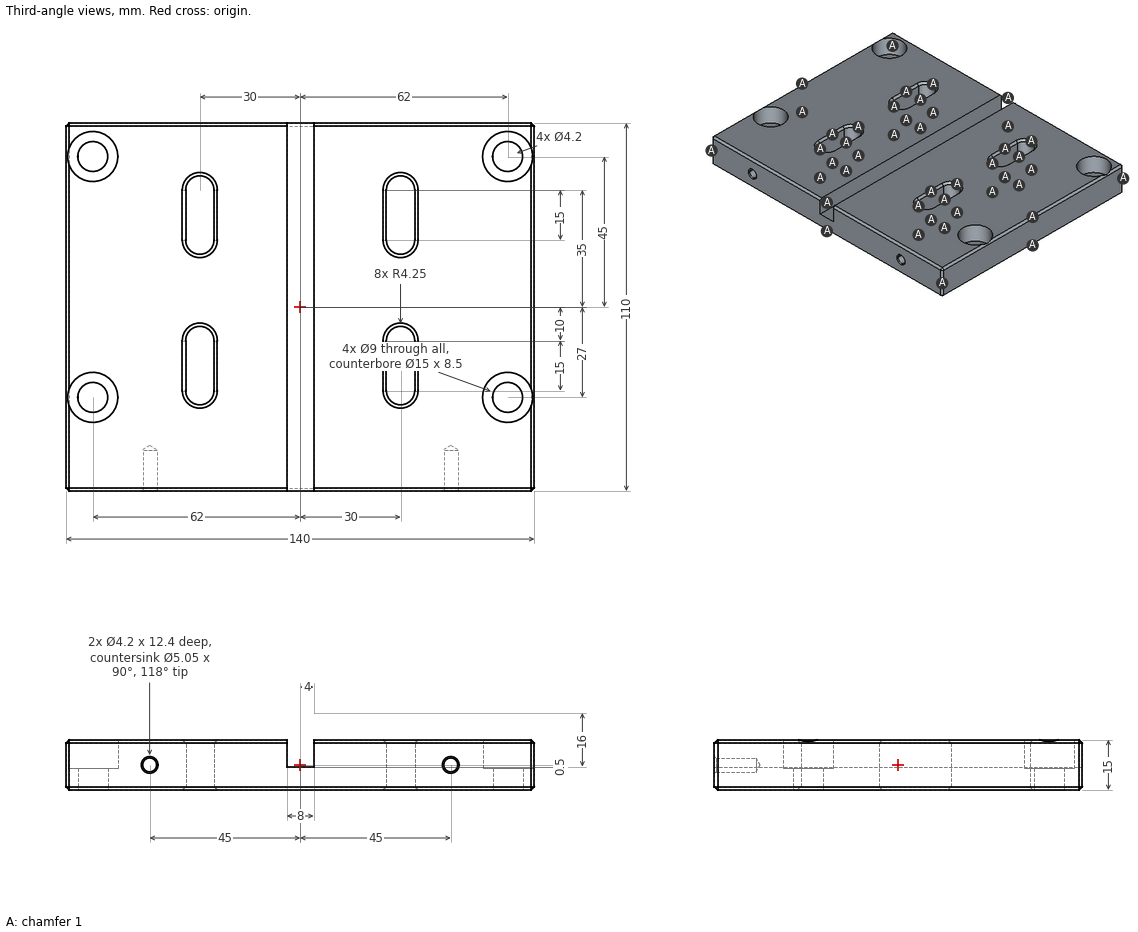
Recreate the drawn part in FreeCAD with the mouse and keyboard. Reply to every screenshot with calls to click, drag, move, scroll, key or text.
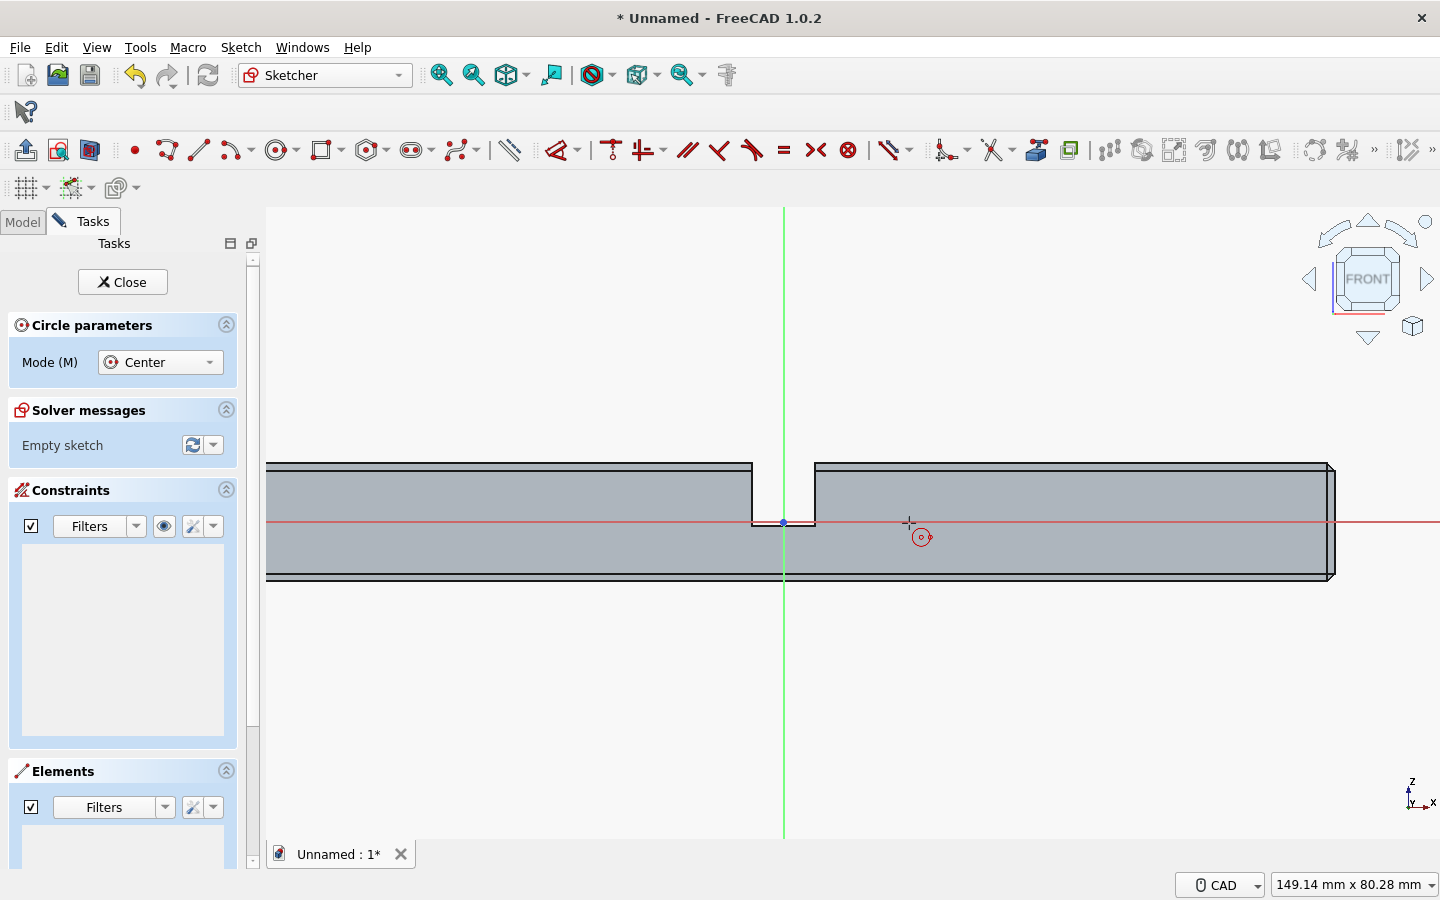
scroll(429, 522, up, 2)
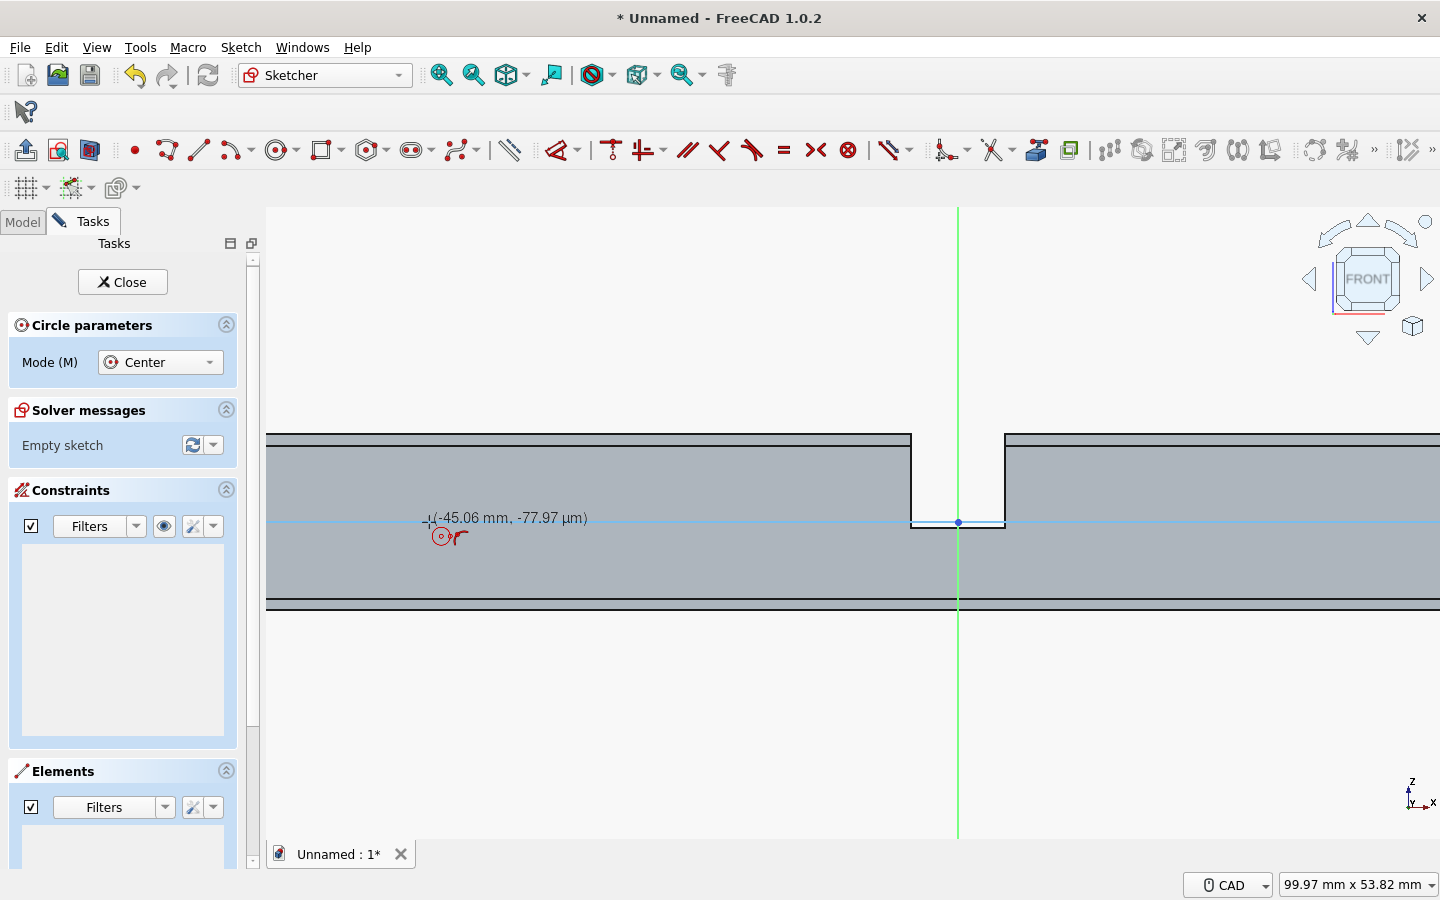
click(430, 522)
click(447, 505)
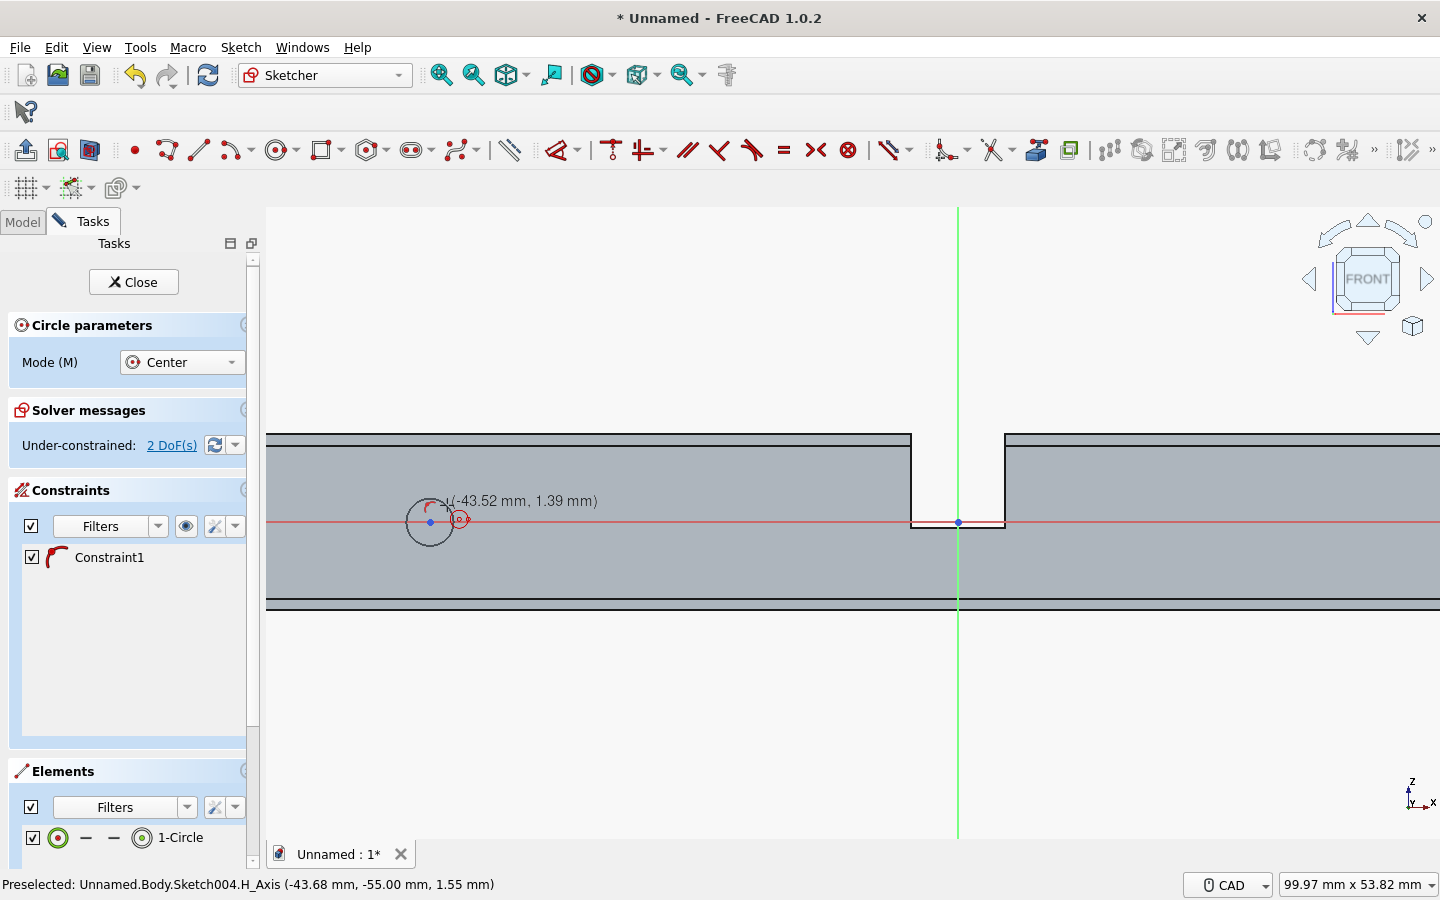
scroll(432, 524, down, 2)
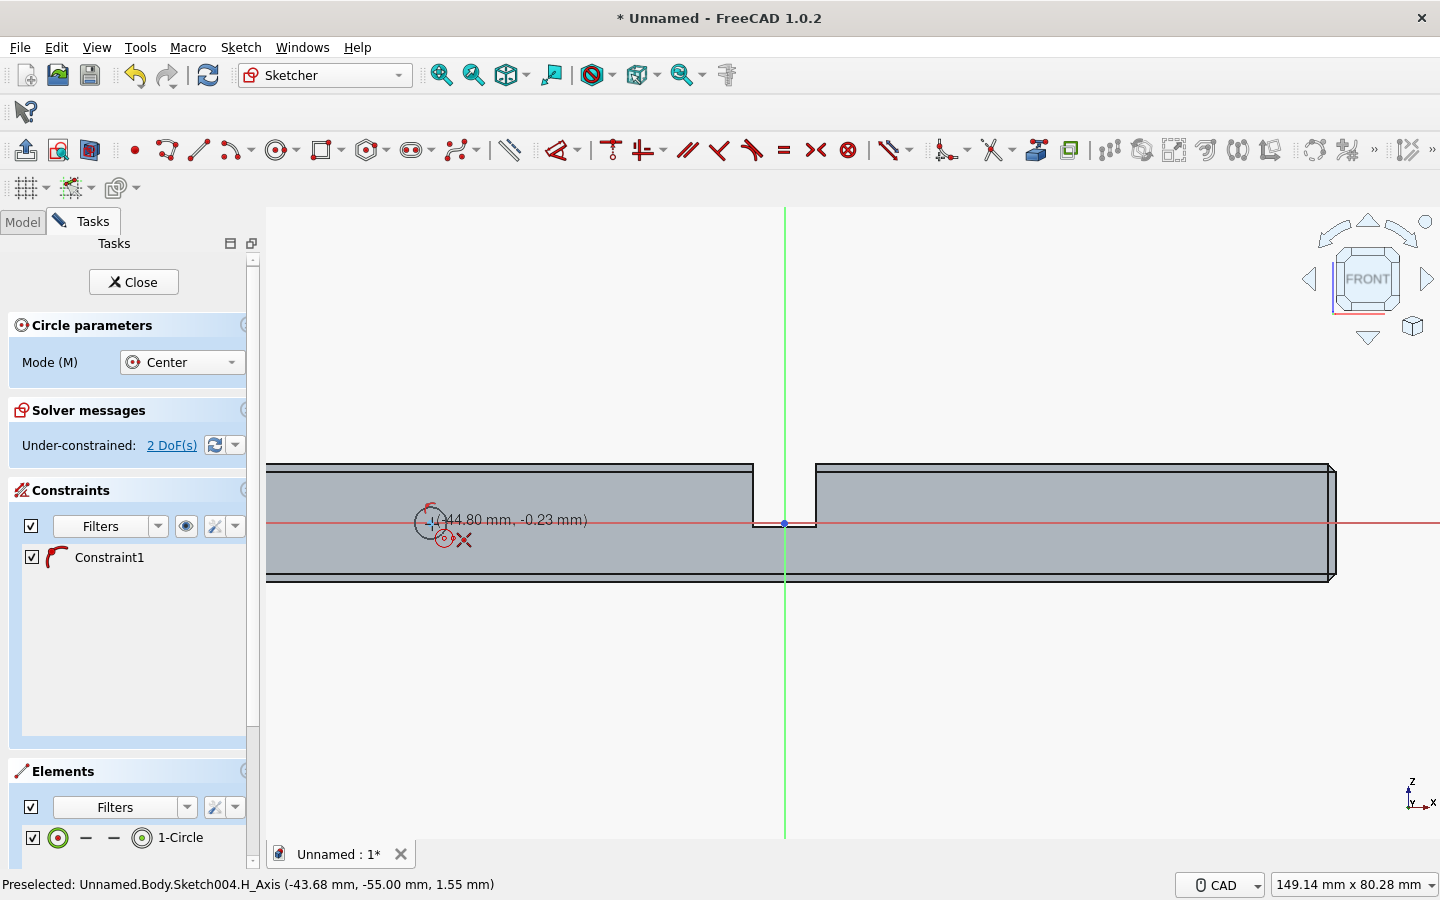
scroll(1139, 523, up, 2)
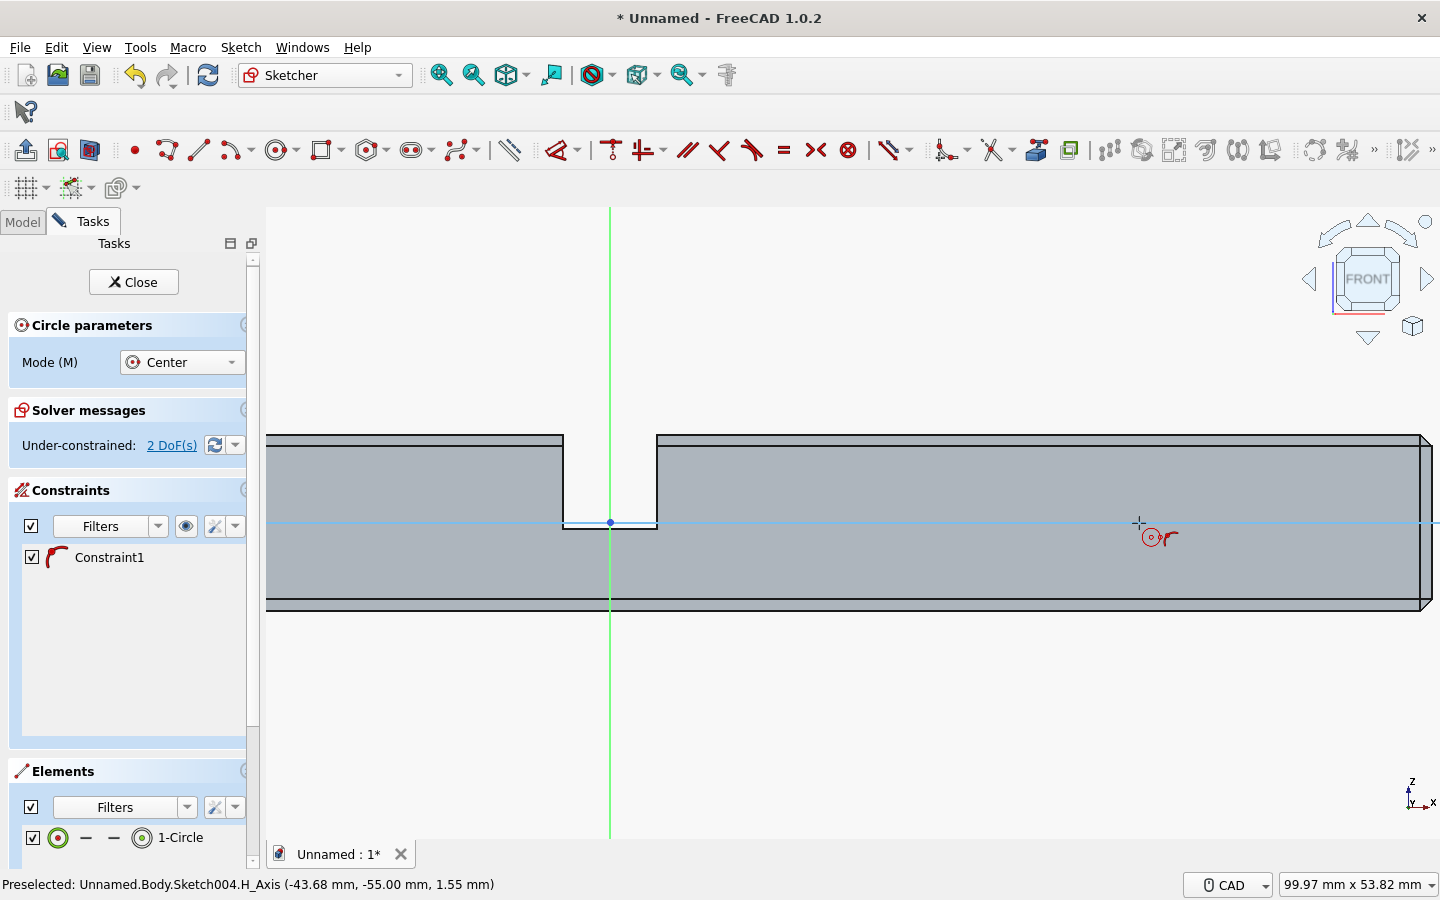
click(1139, 523)
click(1156, 505)
key(Escape)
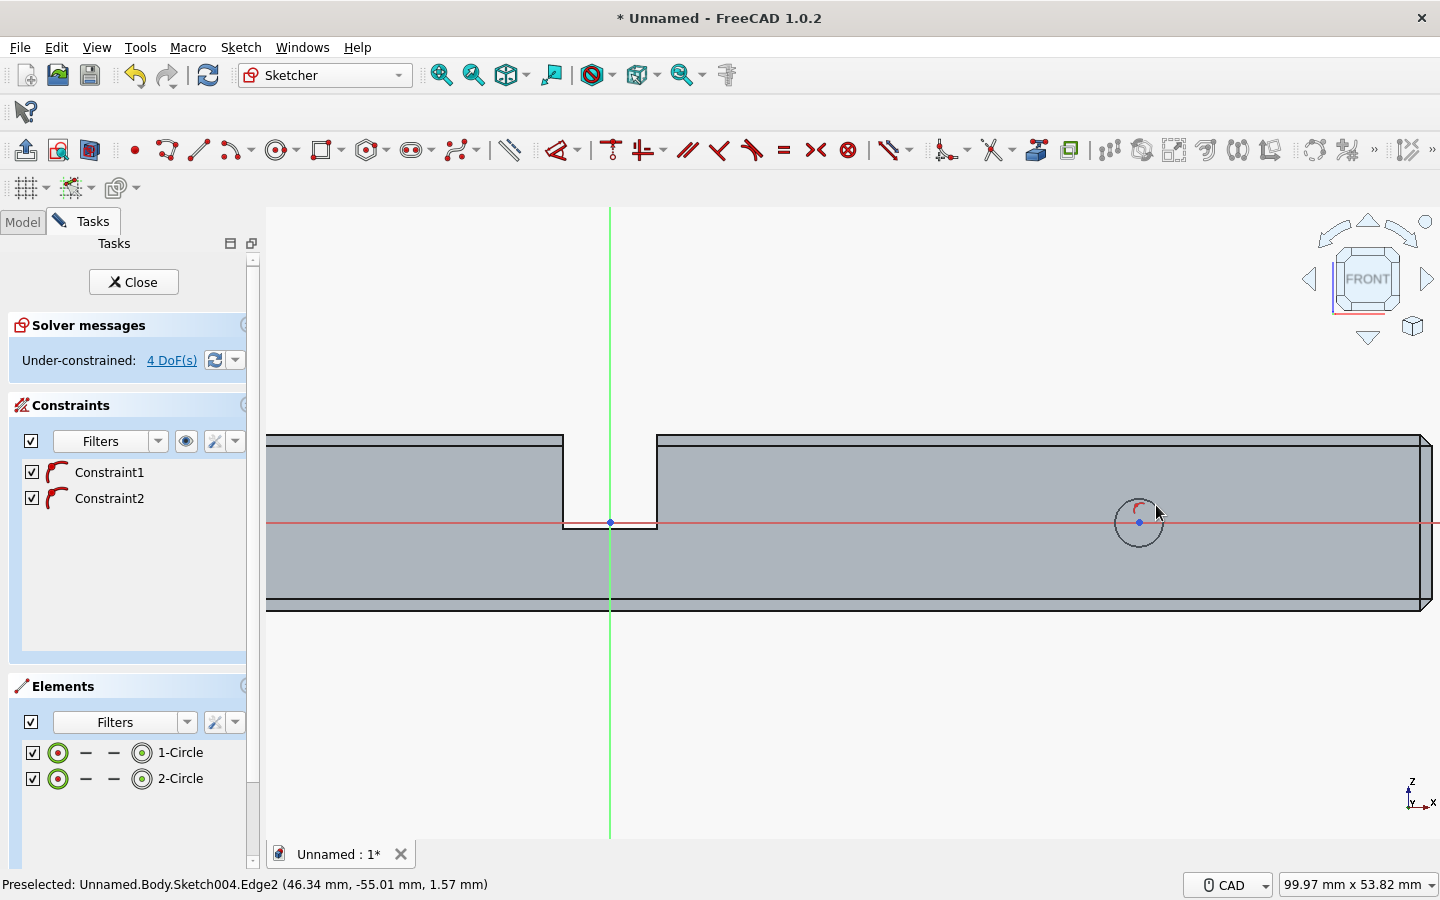
scroll(1139, 523, down, 2)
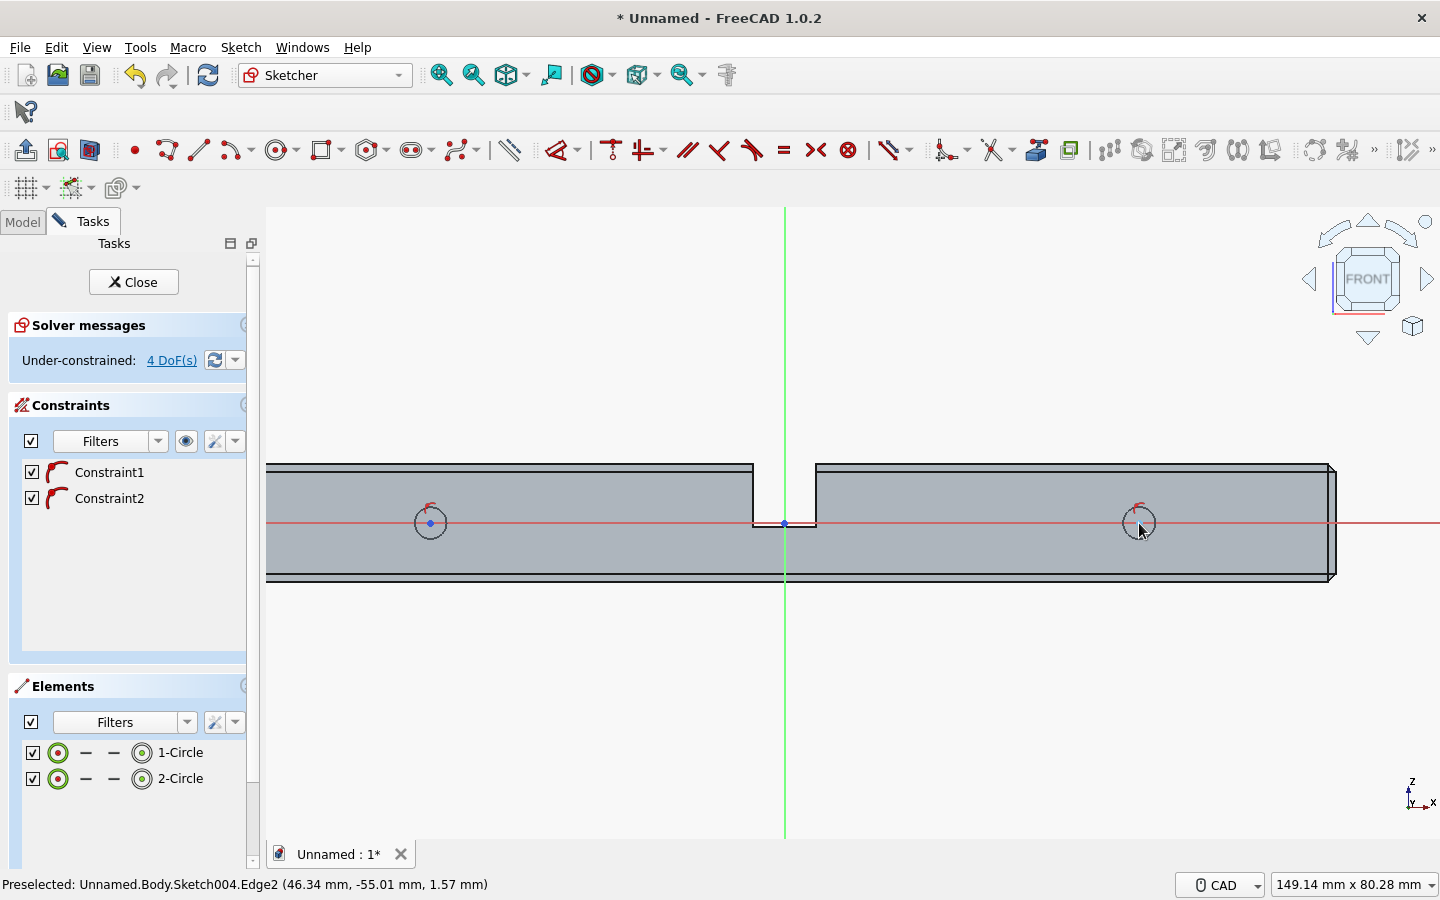
scroll(442, 512, up, 2)